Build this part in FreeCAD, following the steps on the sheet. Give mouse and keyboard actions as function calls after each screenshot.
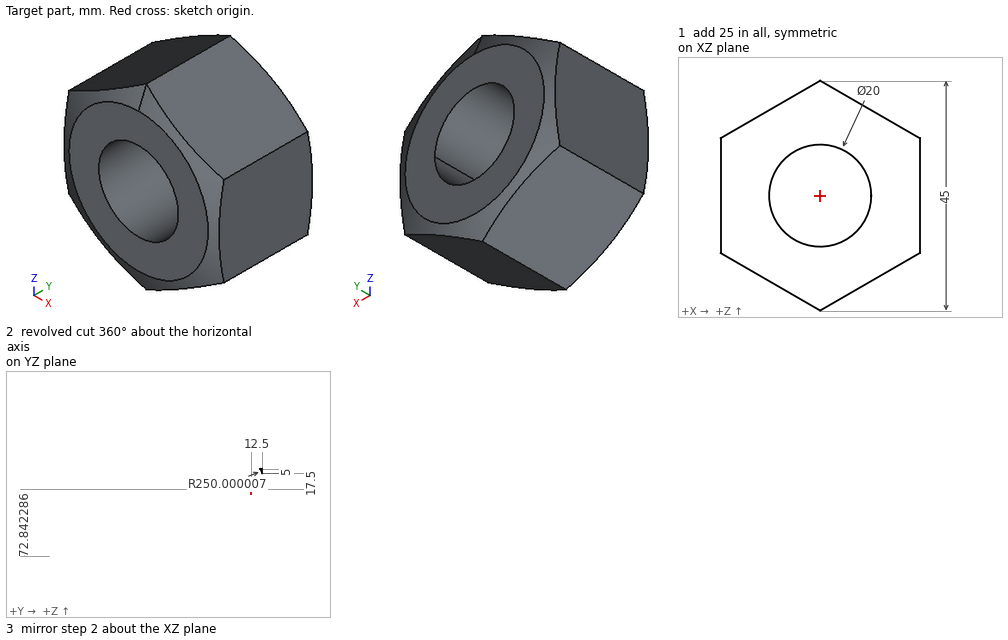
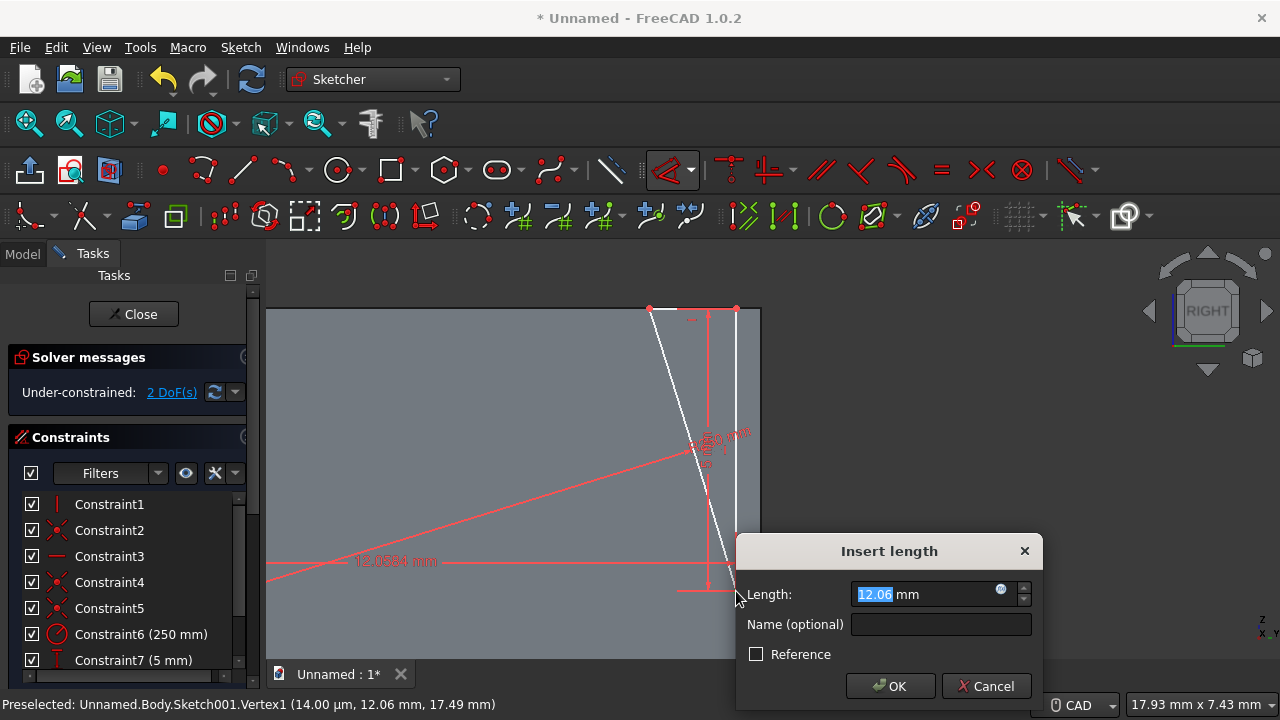
text(12.5)
key(Return)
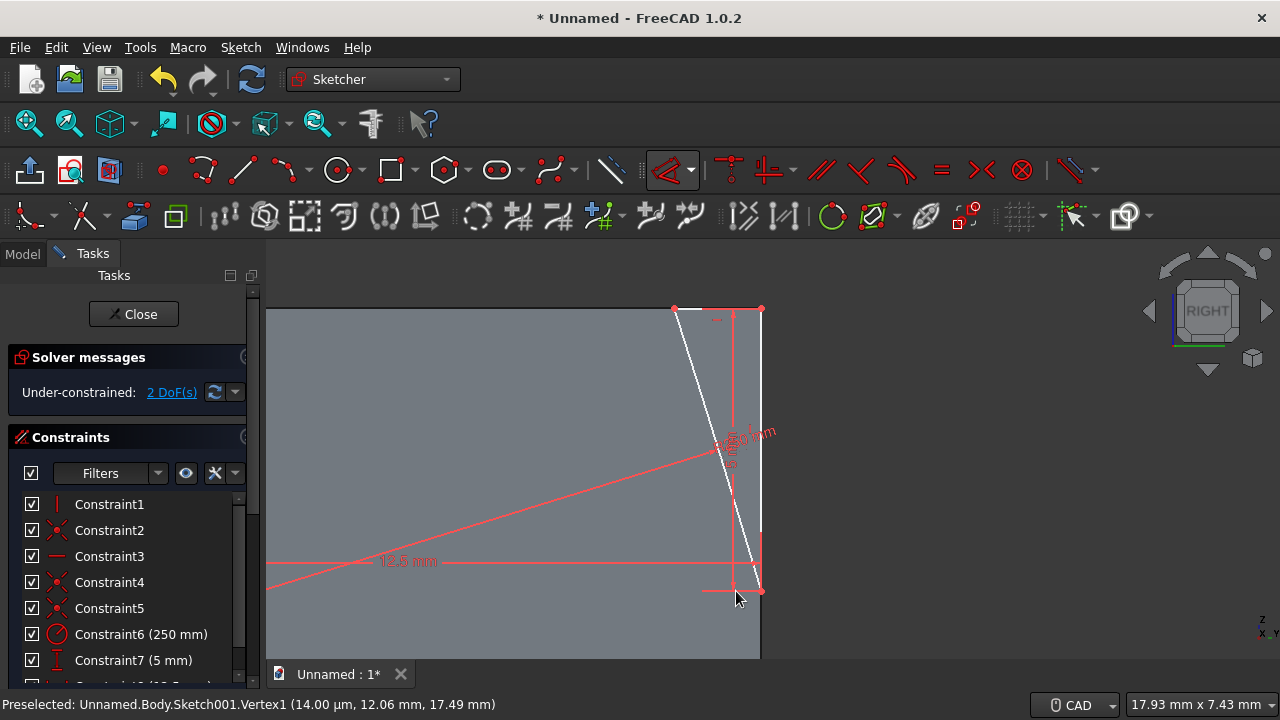
click(761, 591)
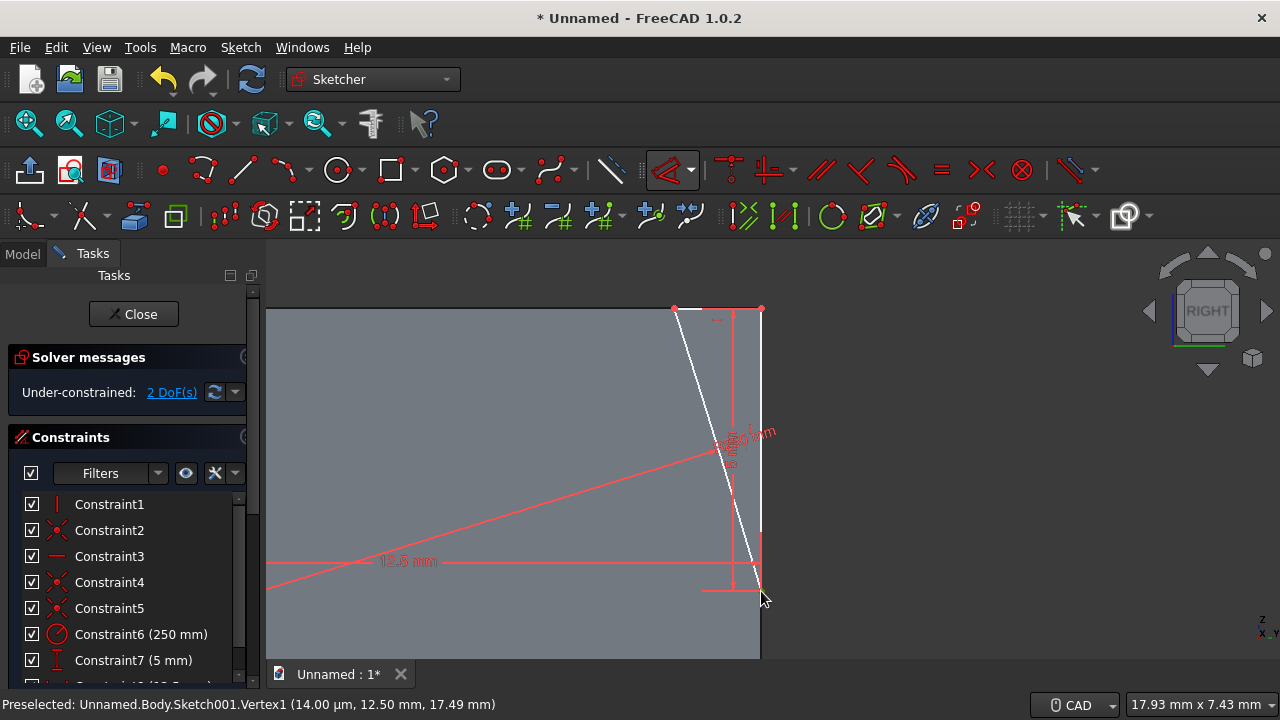
key(i)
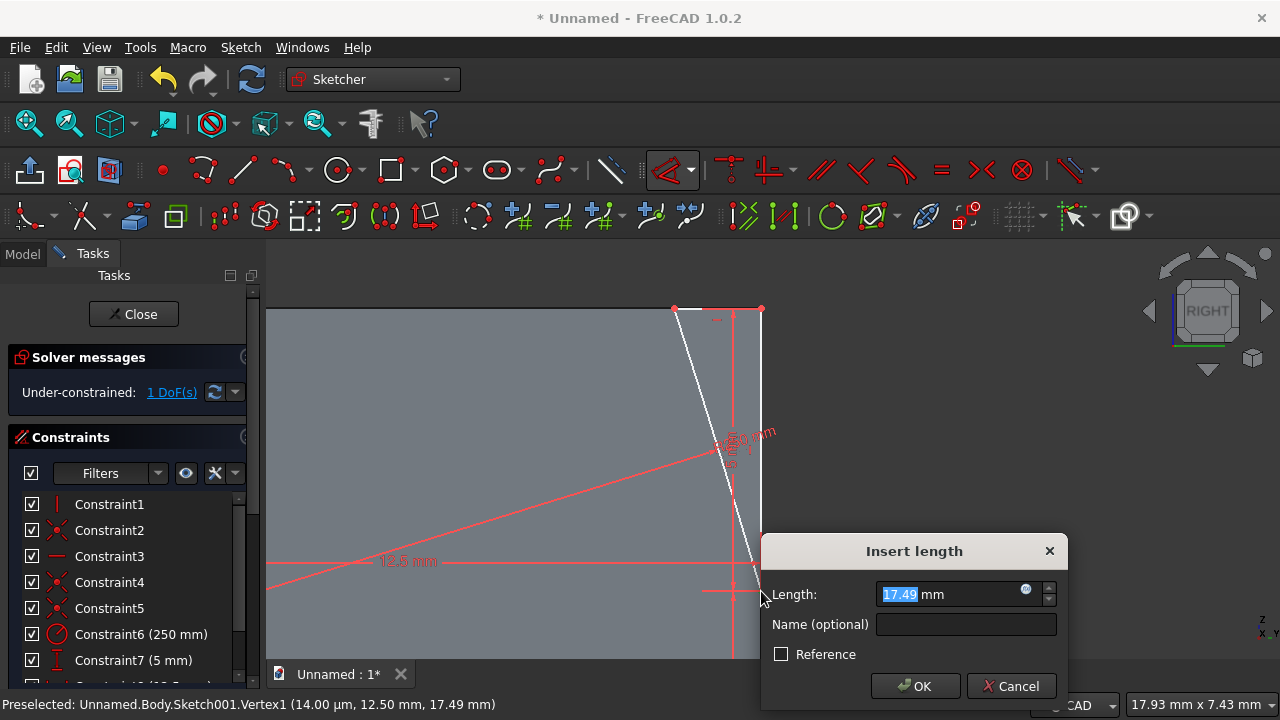
text(17.5)
key(Return)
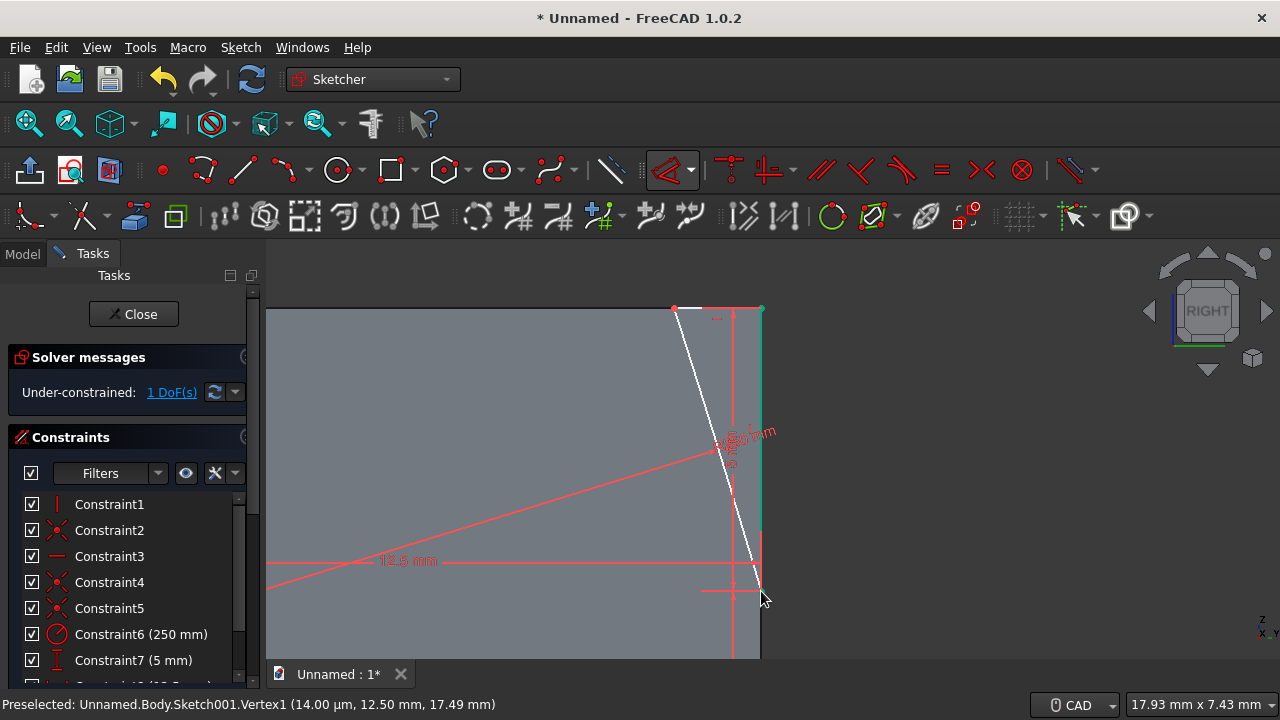
scroll(1057, 343, down, 15)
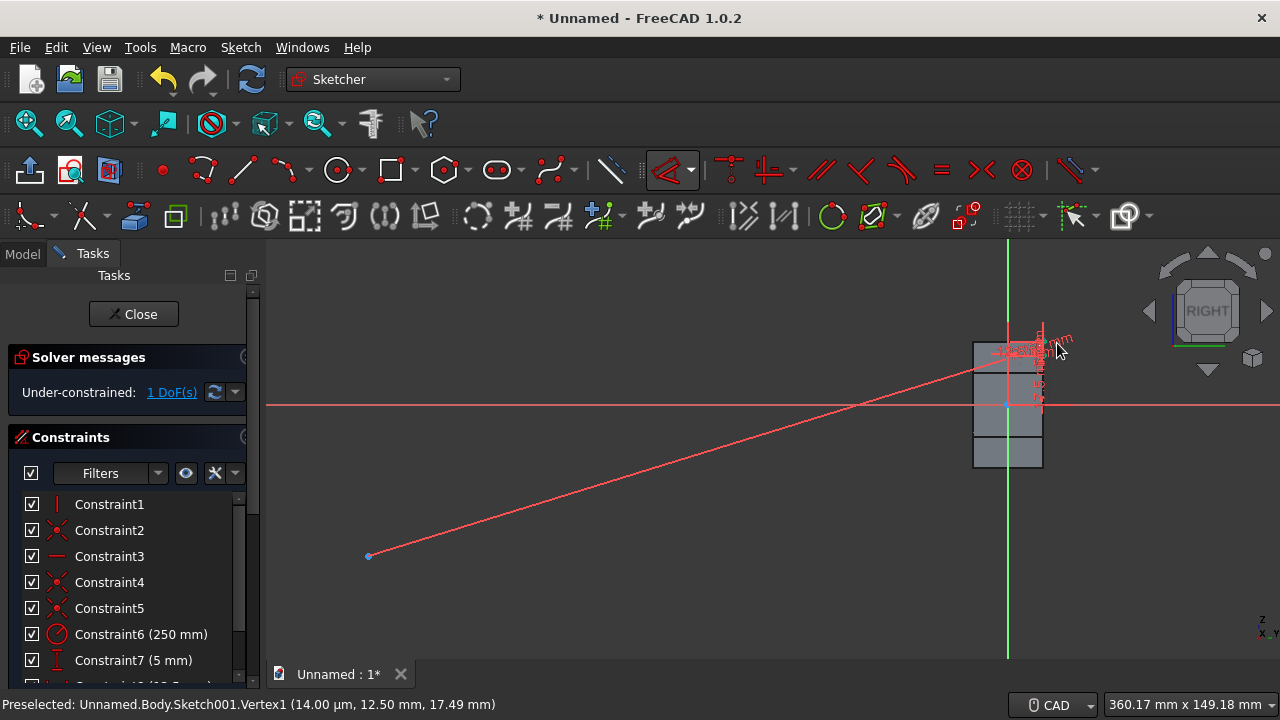
click(368, 556)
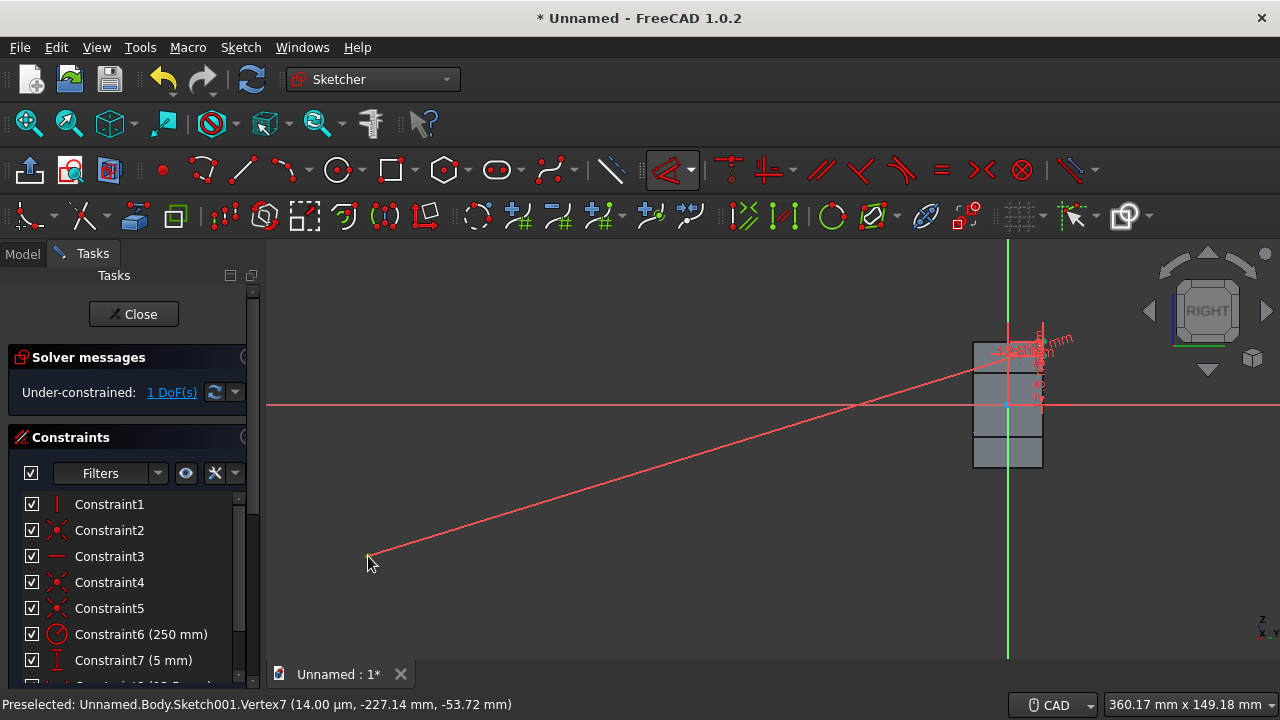
key(i)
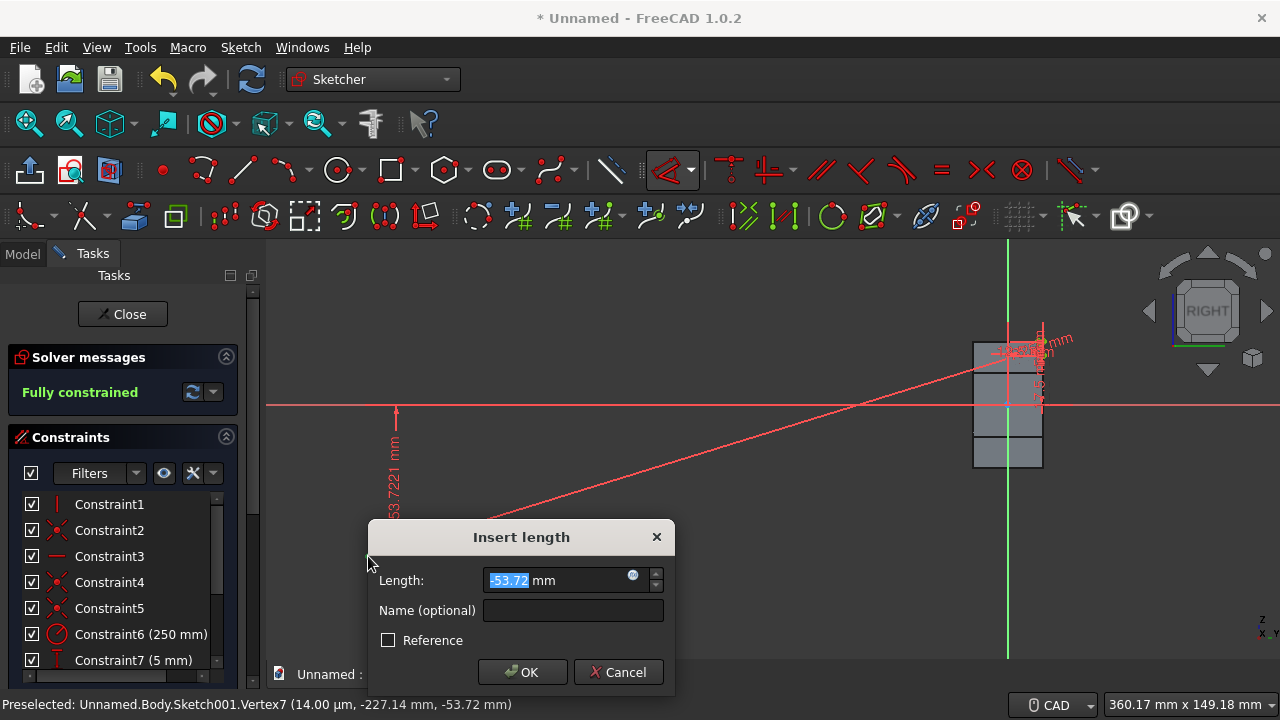
text(-72.842286)
key(Return)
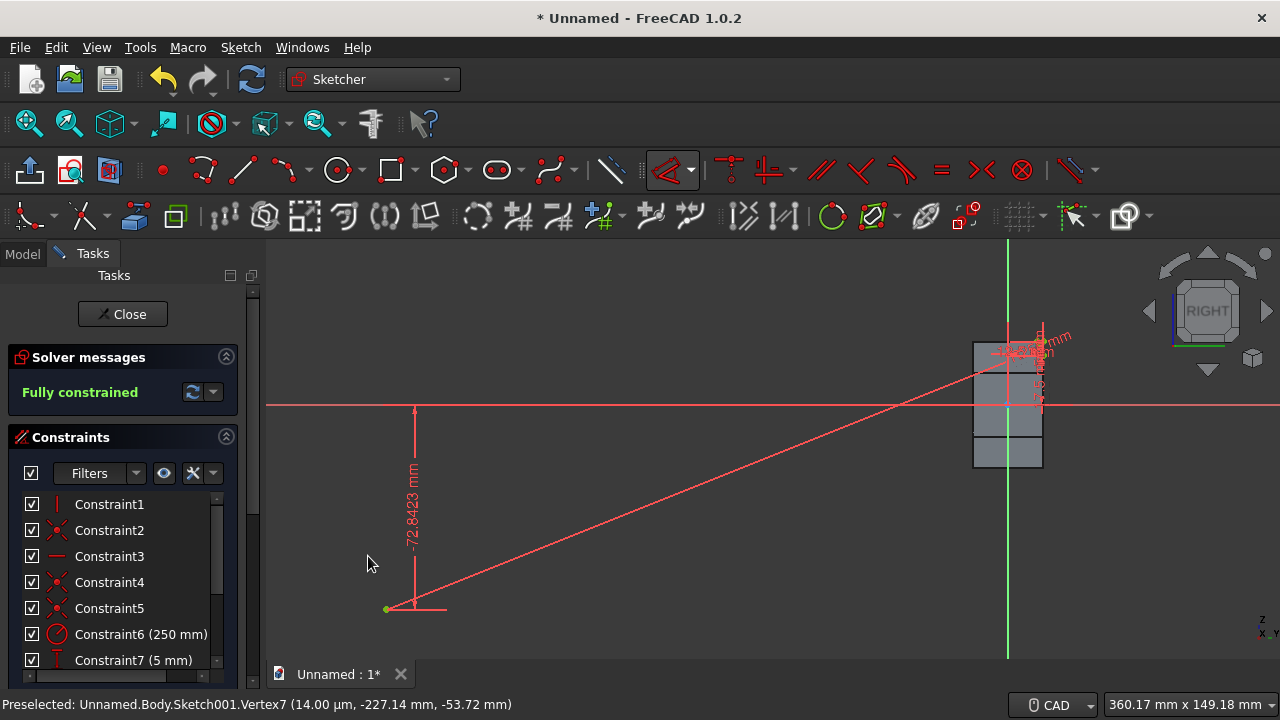
click(123, 314)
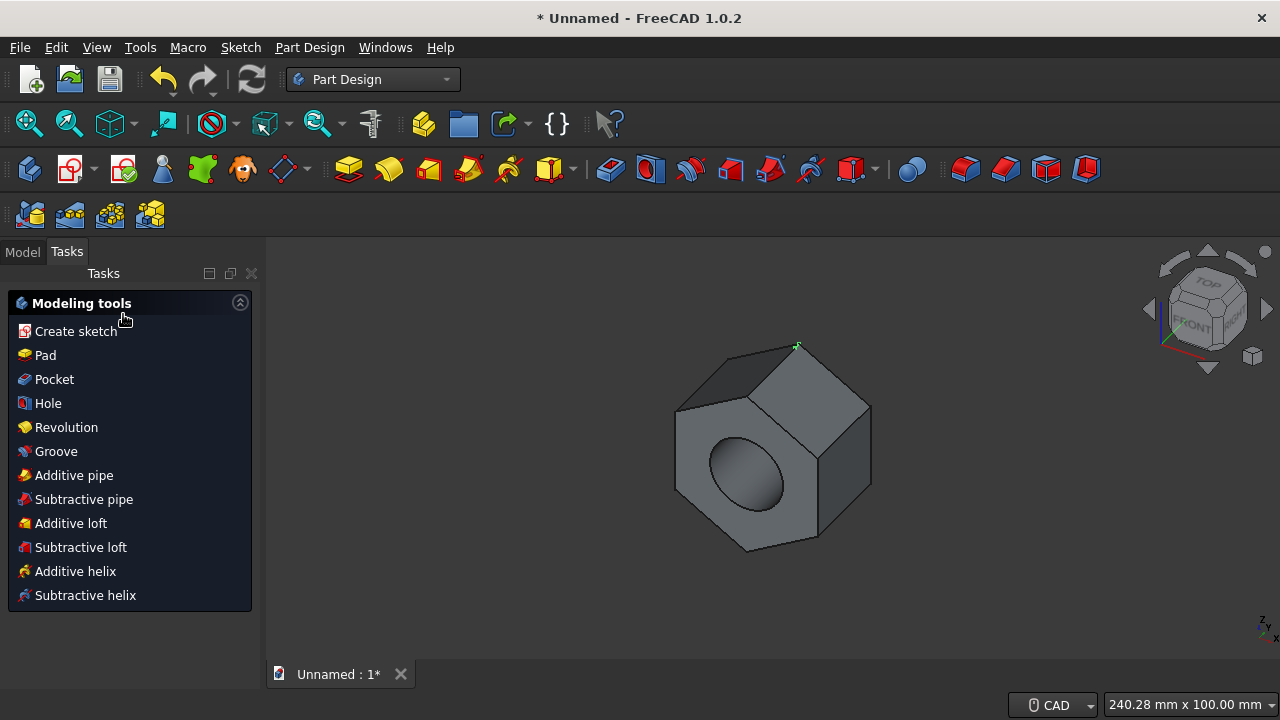
click(692, 170)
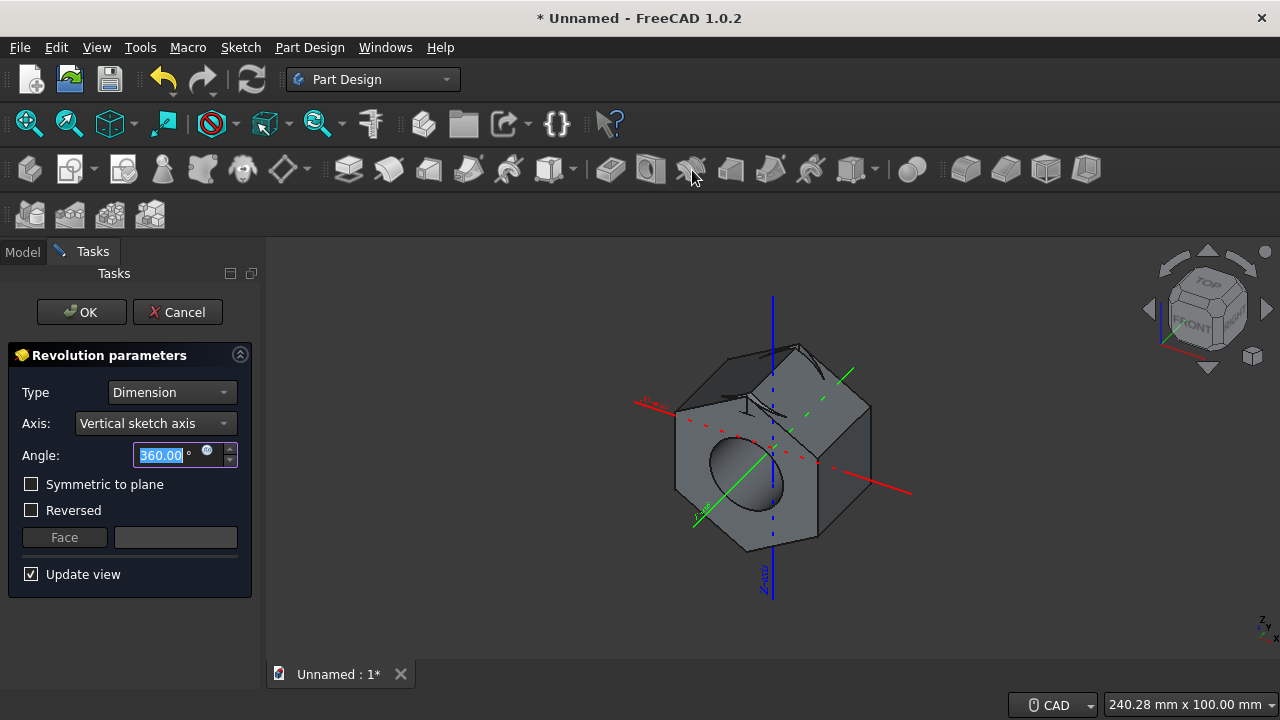
click(156, 424)